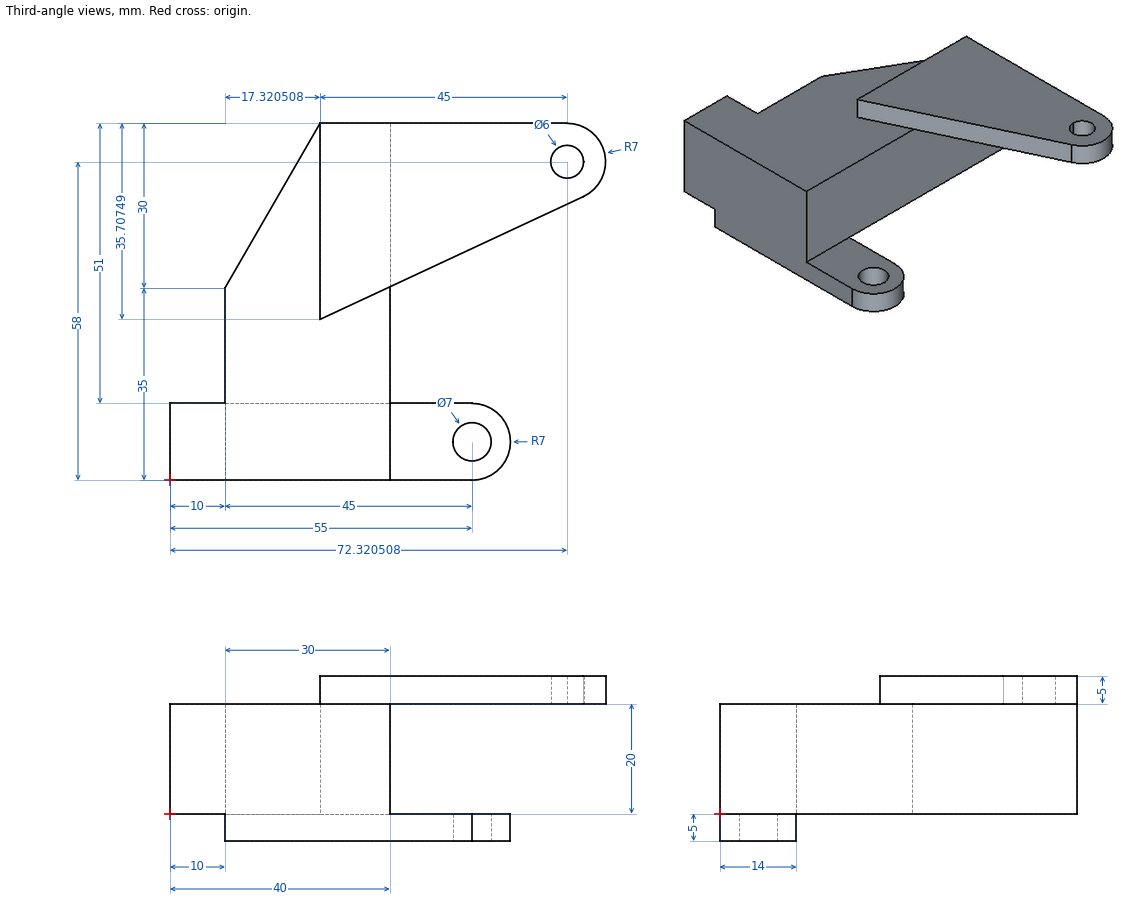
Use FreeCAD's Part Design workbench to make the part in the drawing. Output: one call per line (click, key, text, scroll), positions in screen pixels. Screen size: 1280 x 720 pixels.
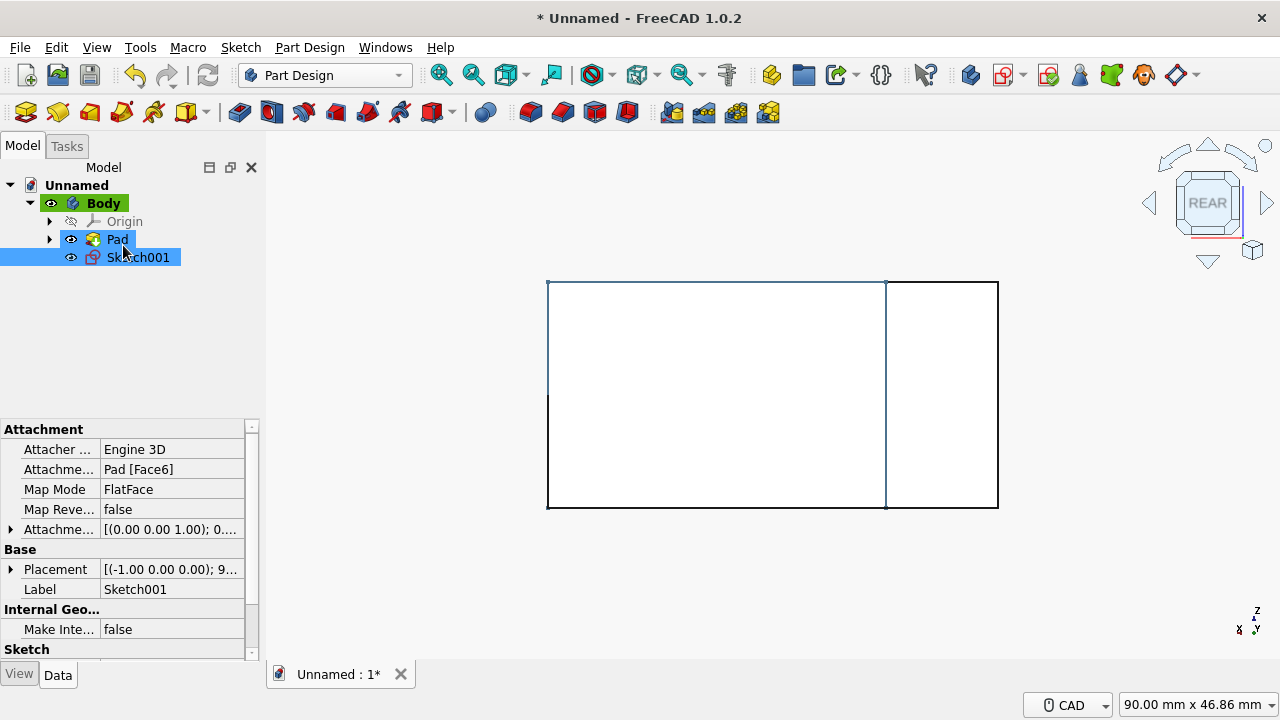
click(26, 112)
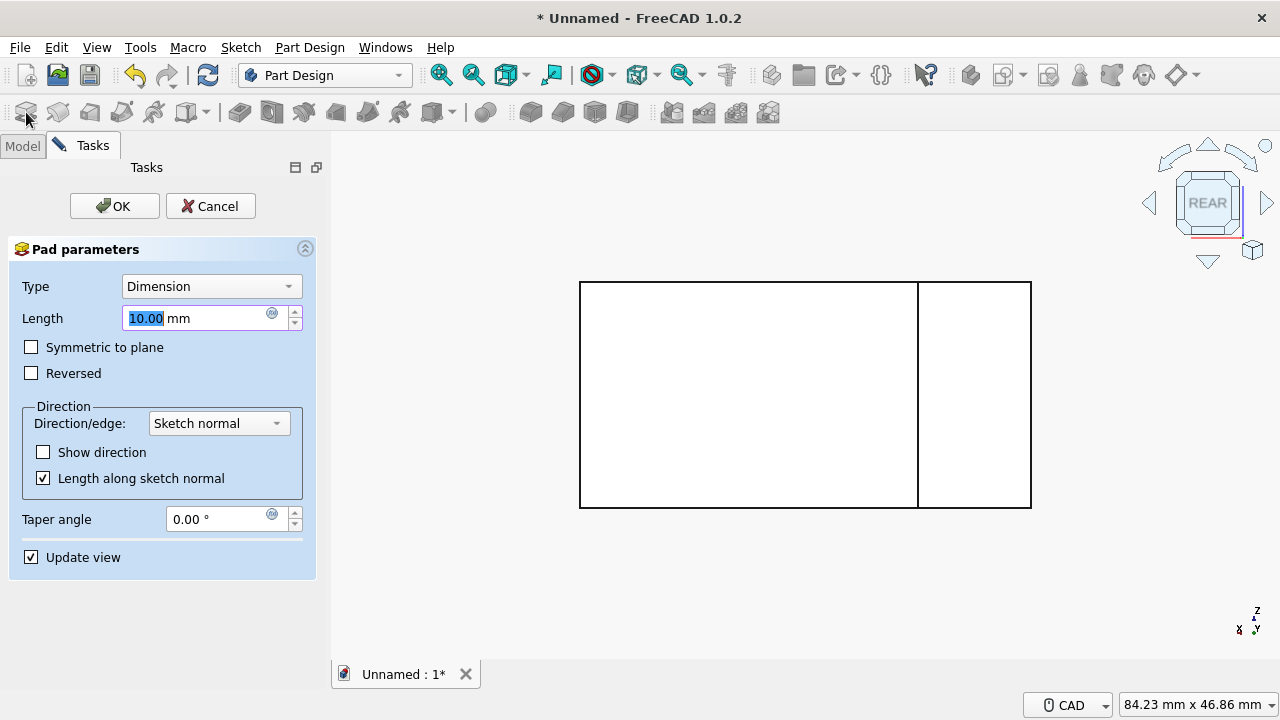
text(51)
key(Tab)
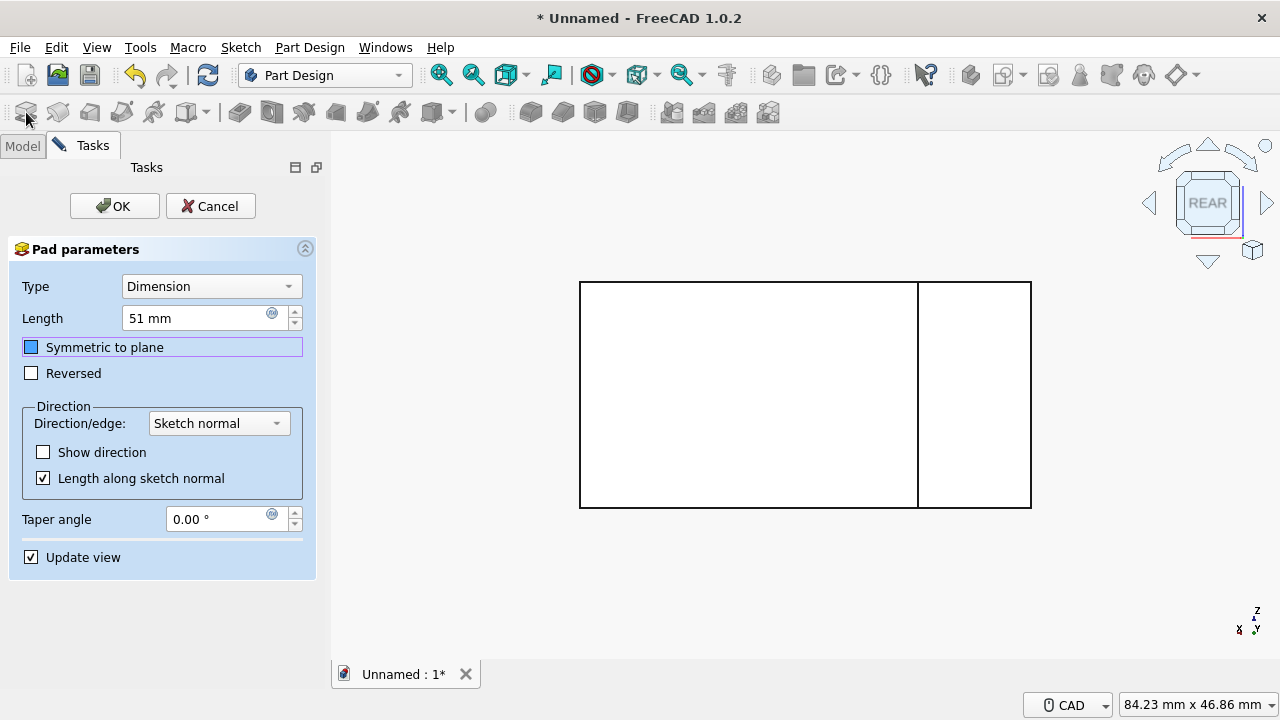
click(115, 206)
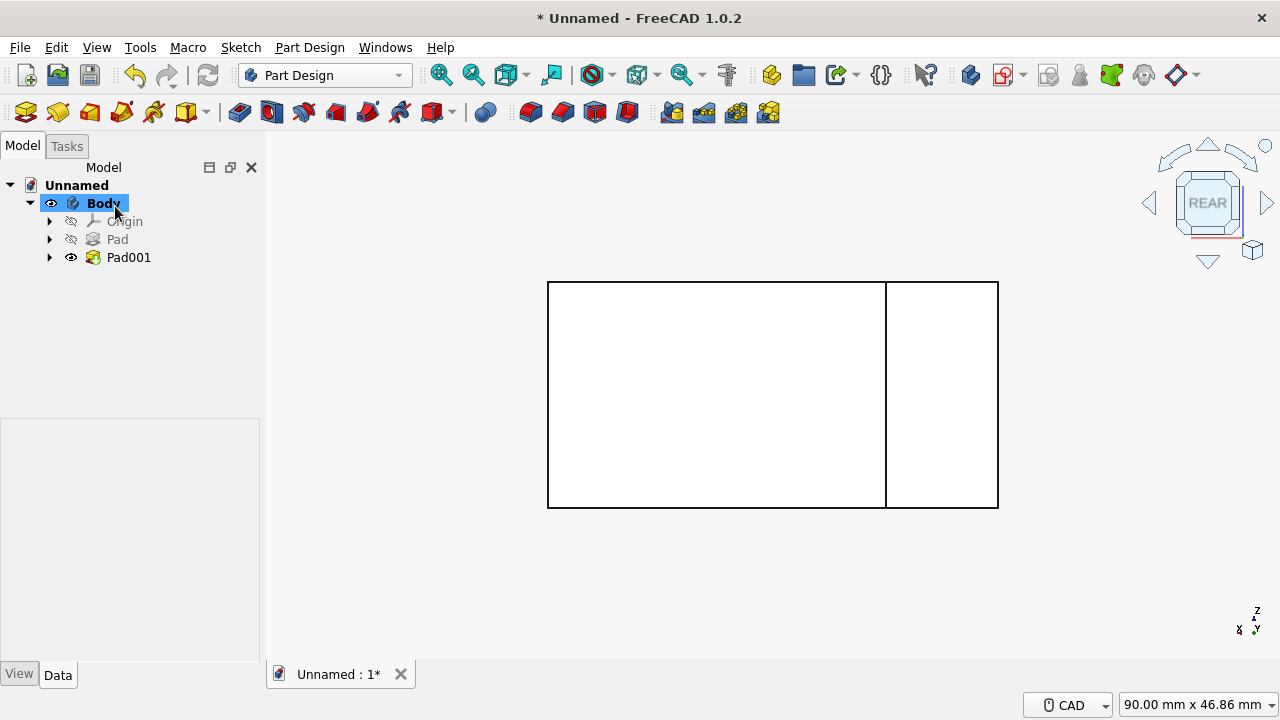
click(442, 76)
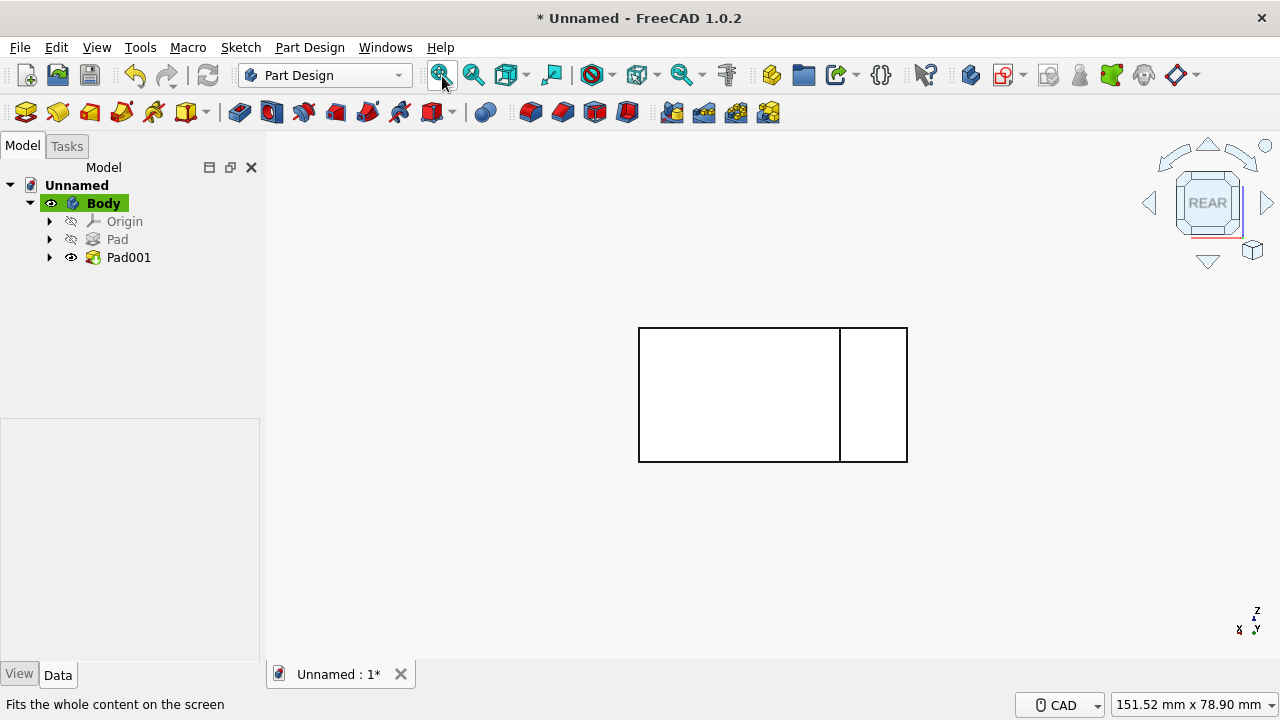
key(0)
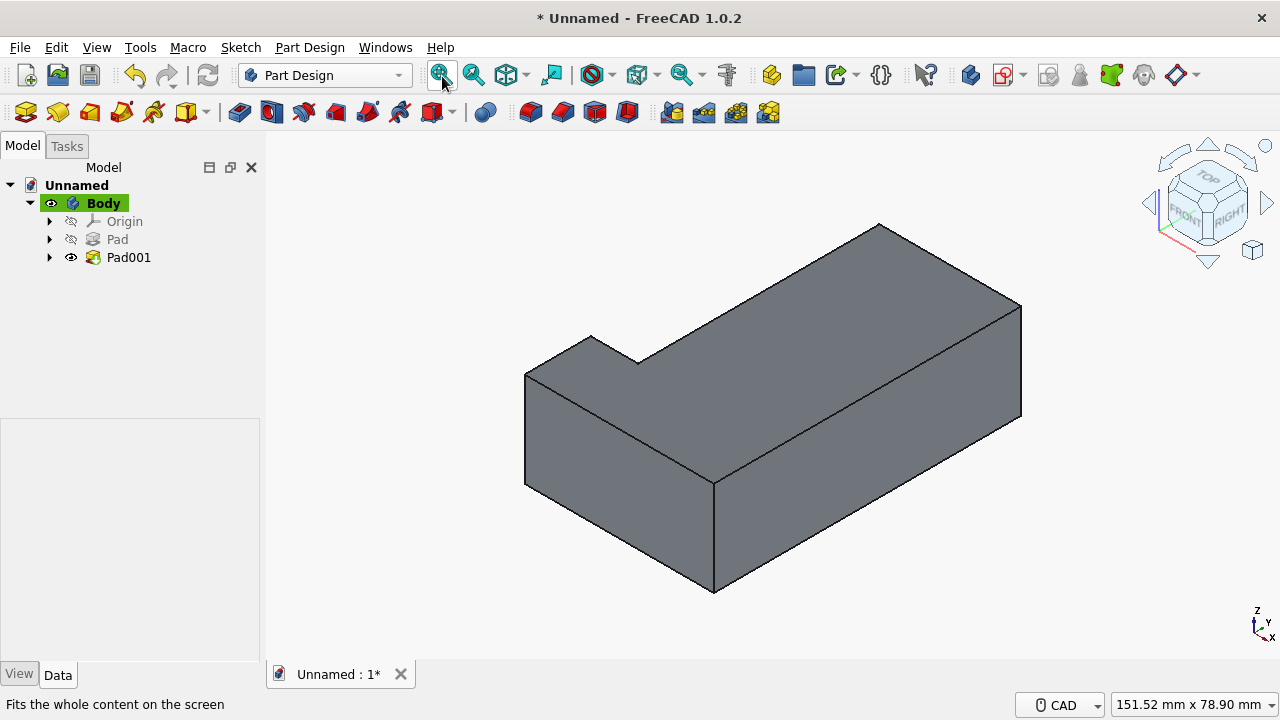
click(844, 330)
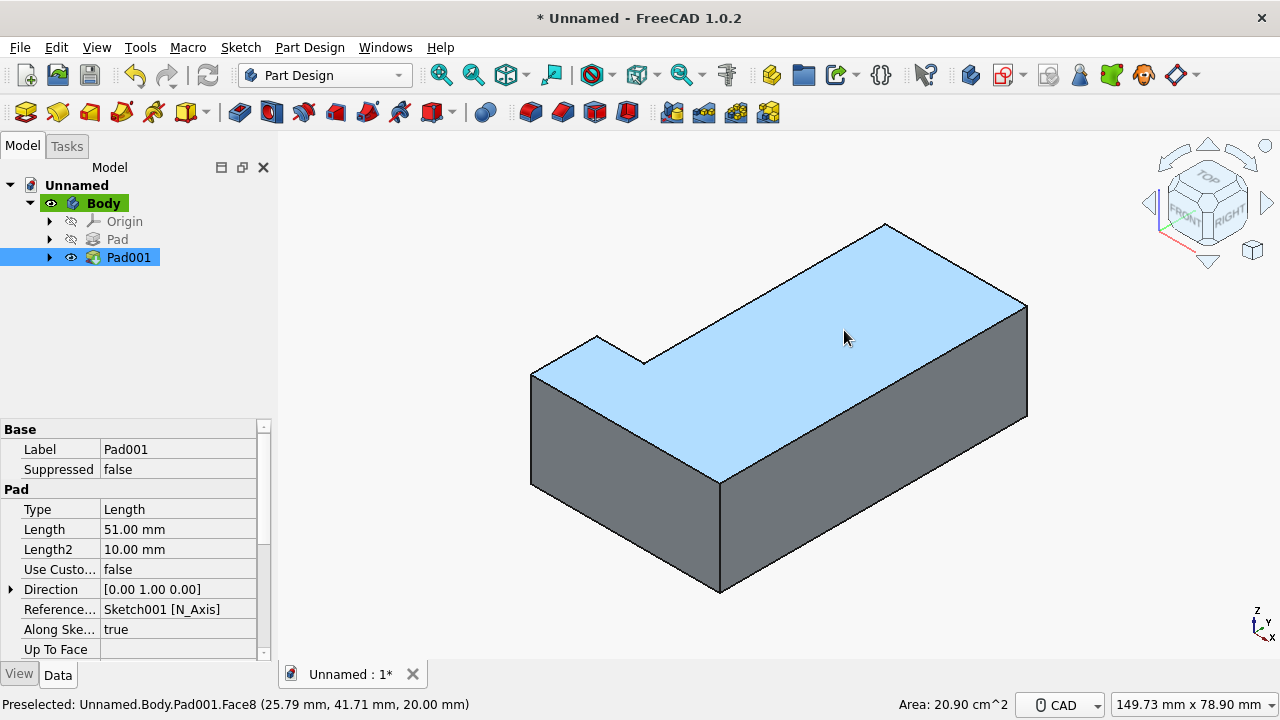
click(1004, 76)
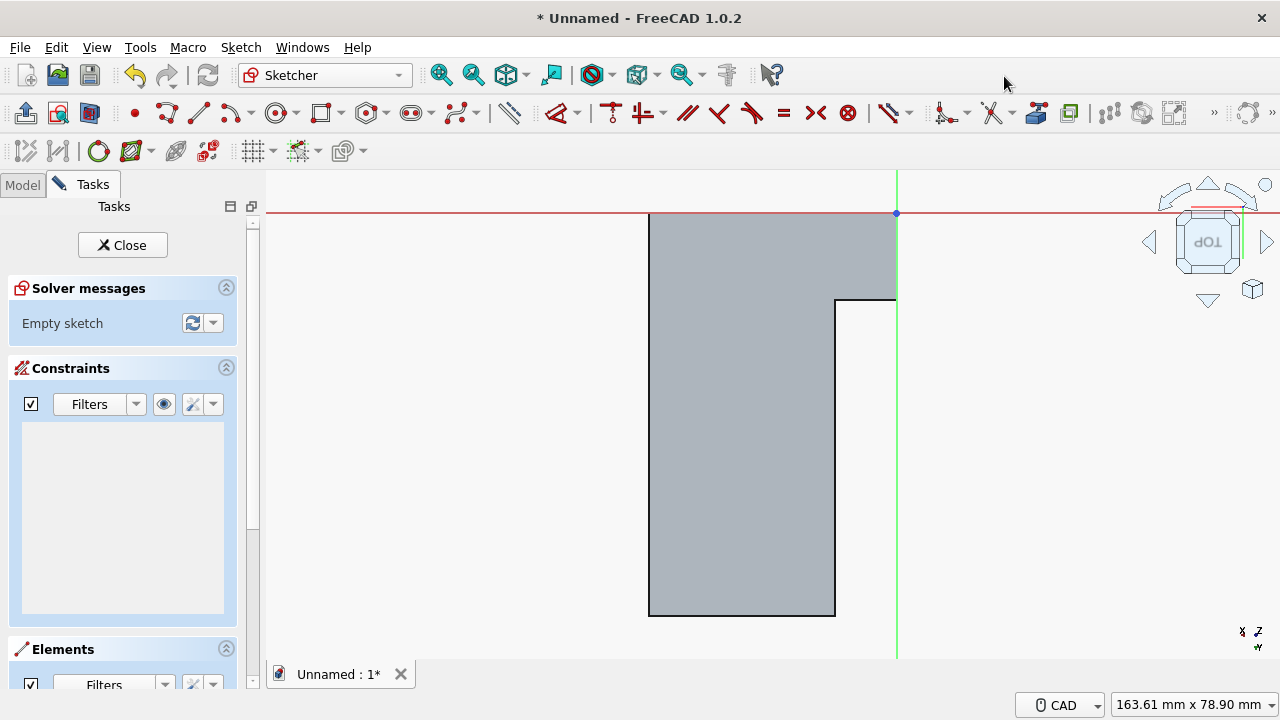
scroll(294, 415, down, 1)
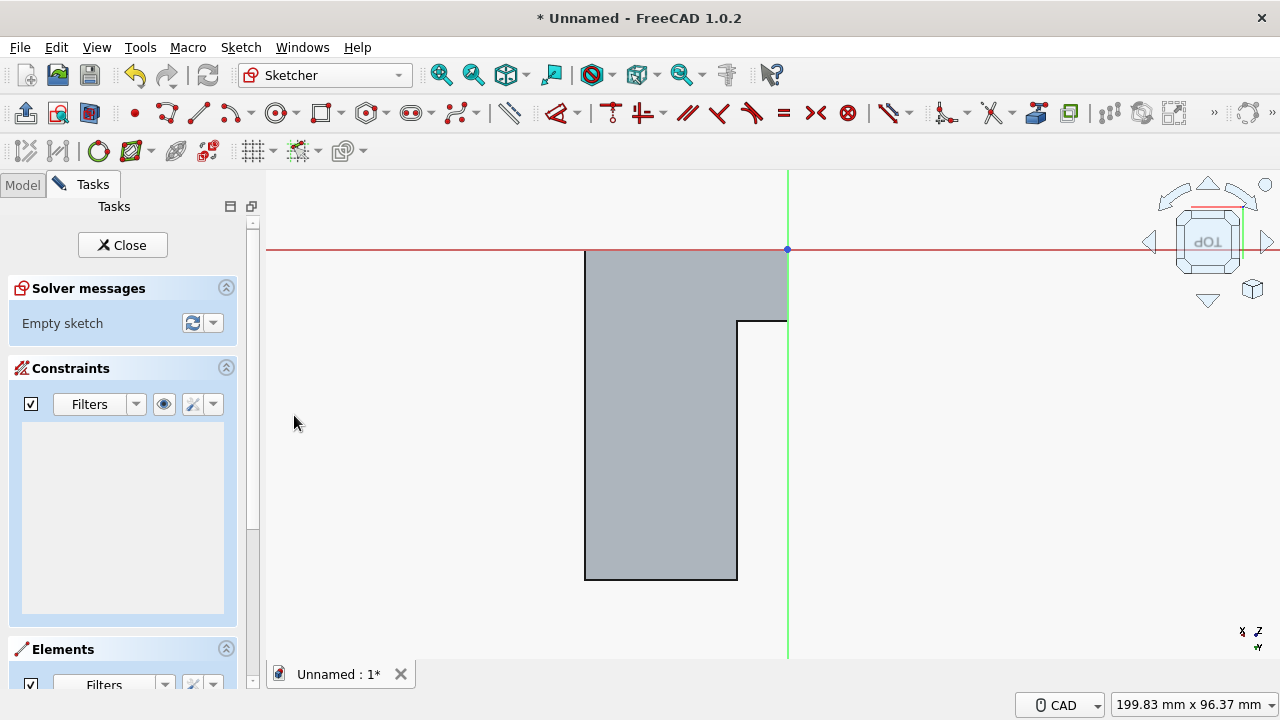
click(168, 114)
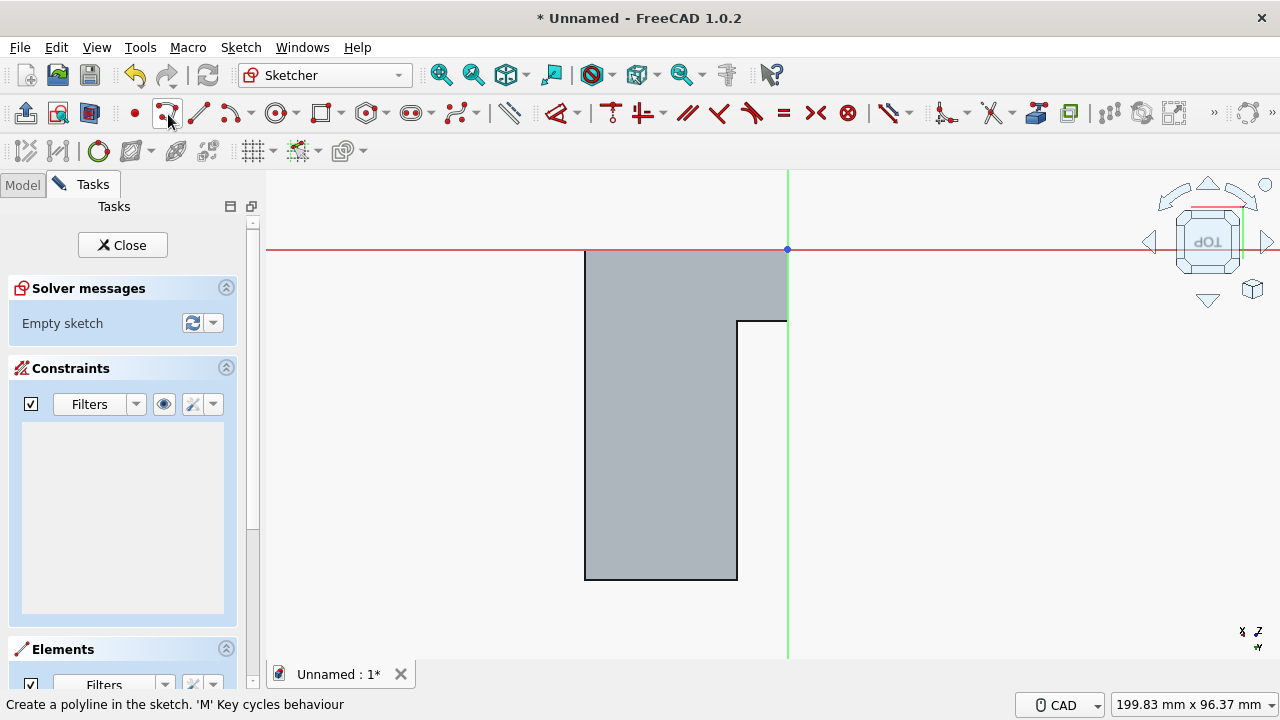
click(737, 427)
click(649, 580)
click(737, 580)
click(737, 428)
key(Escape)
key(Escape)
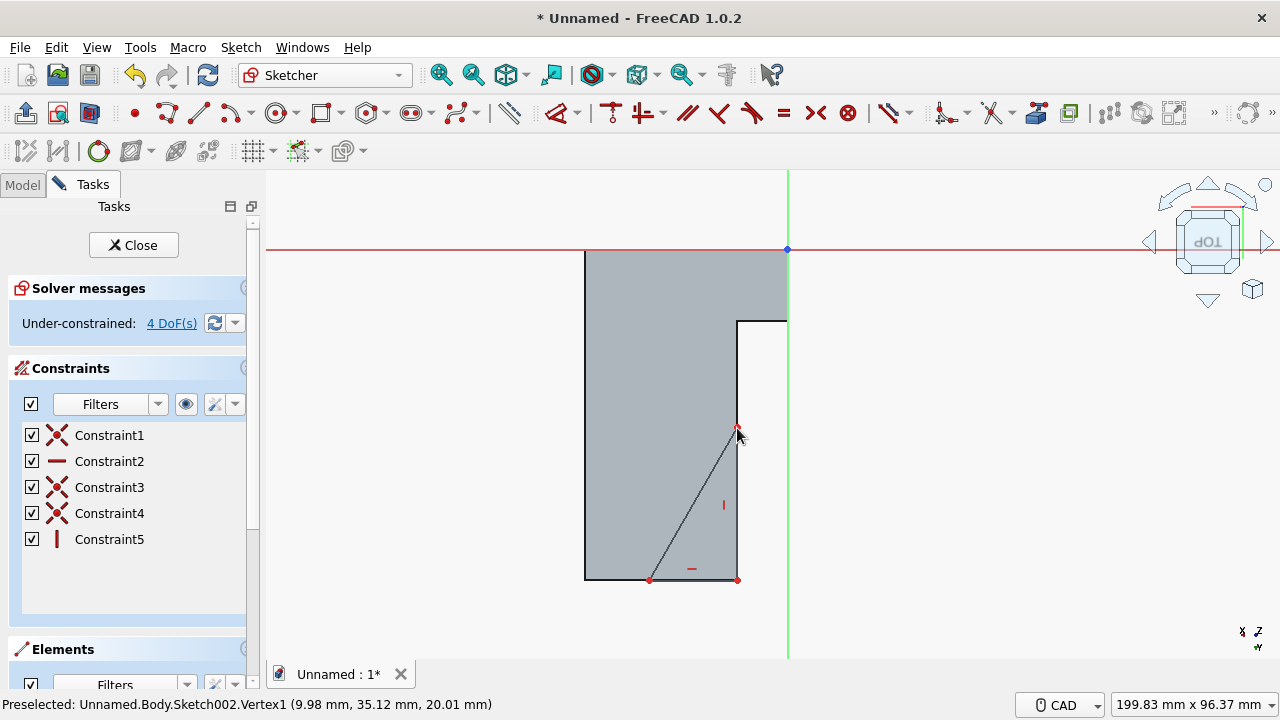
click(556, 114)